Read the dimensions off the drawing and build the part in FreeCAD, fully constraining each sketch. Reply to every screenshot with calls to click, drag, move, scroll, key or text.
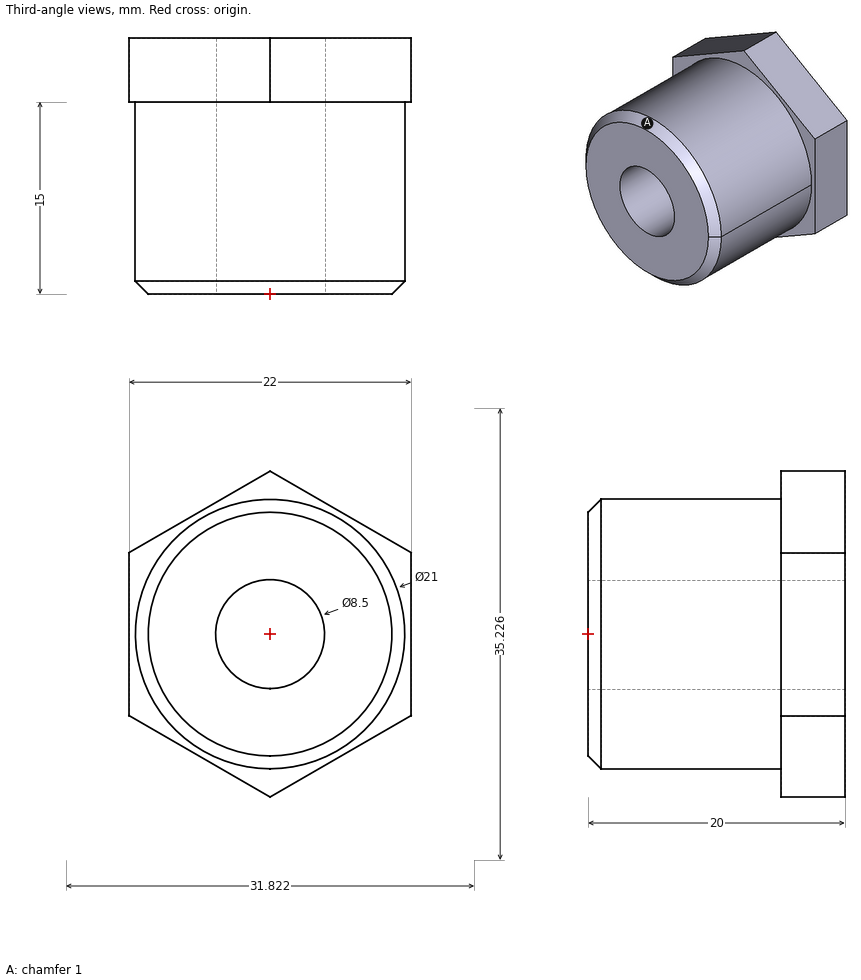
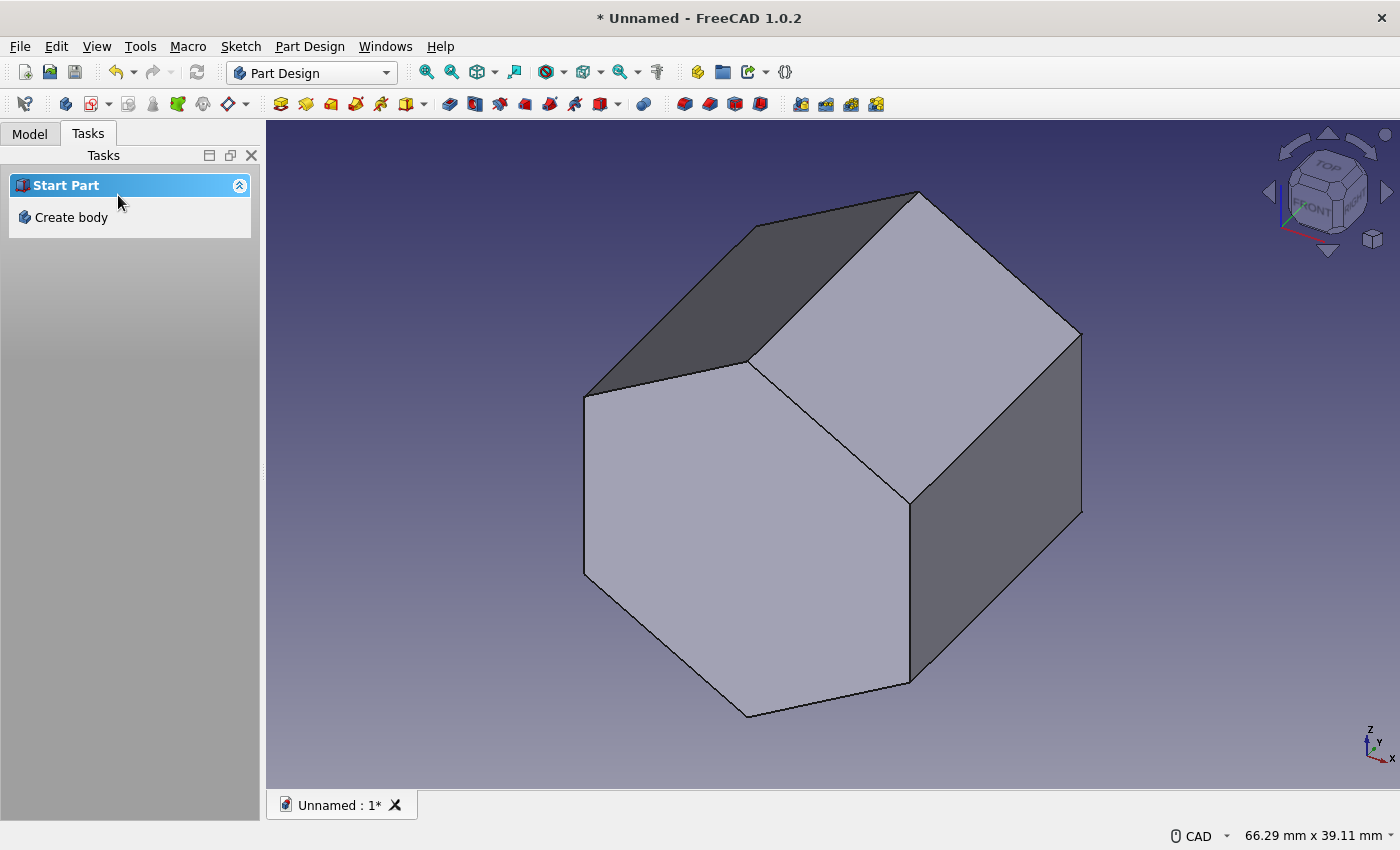
click(747, 538)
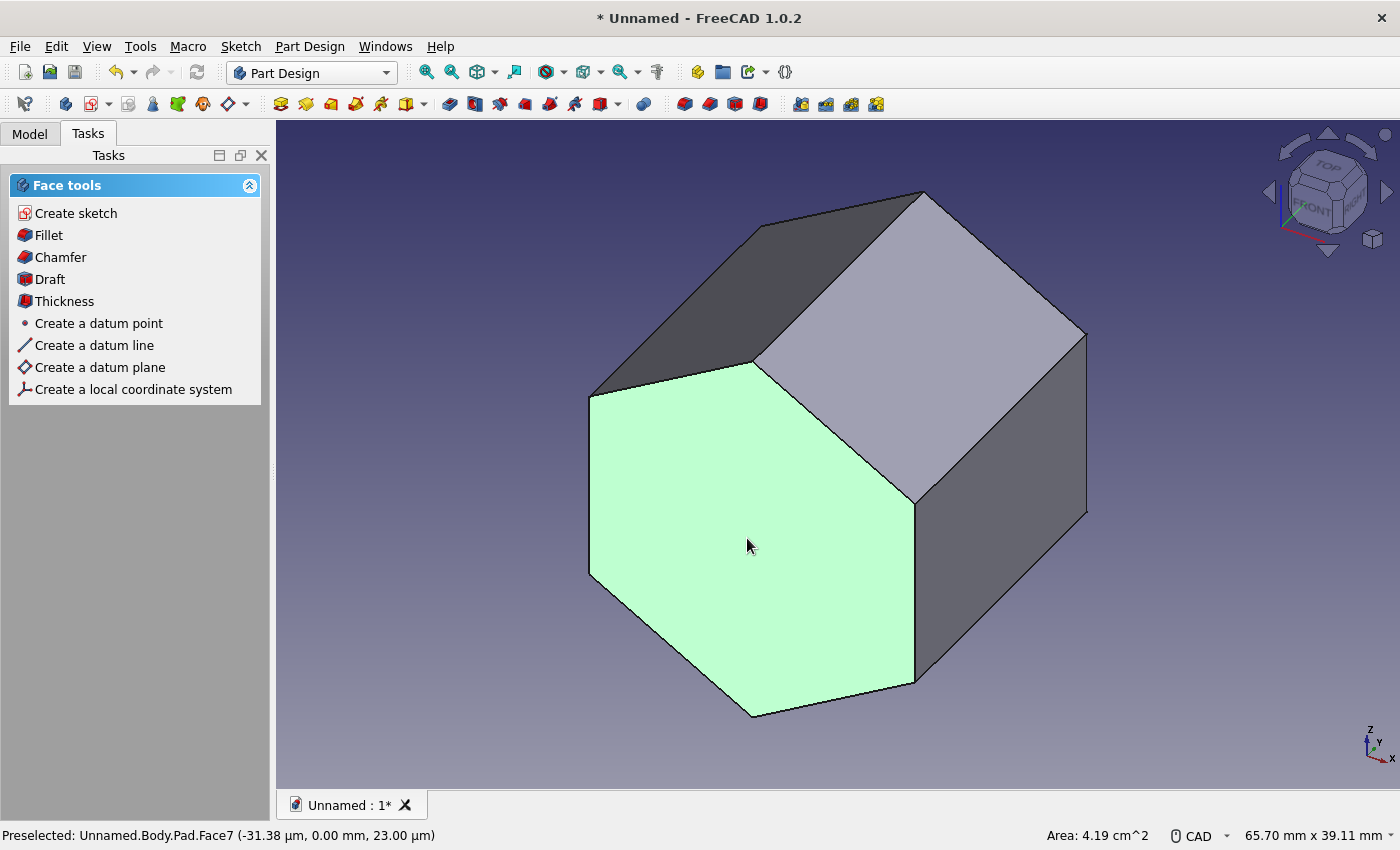
click(90, 104)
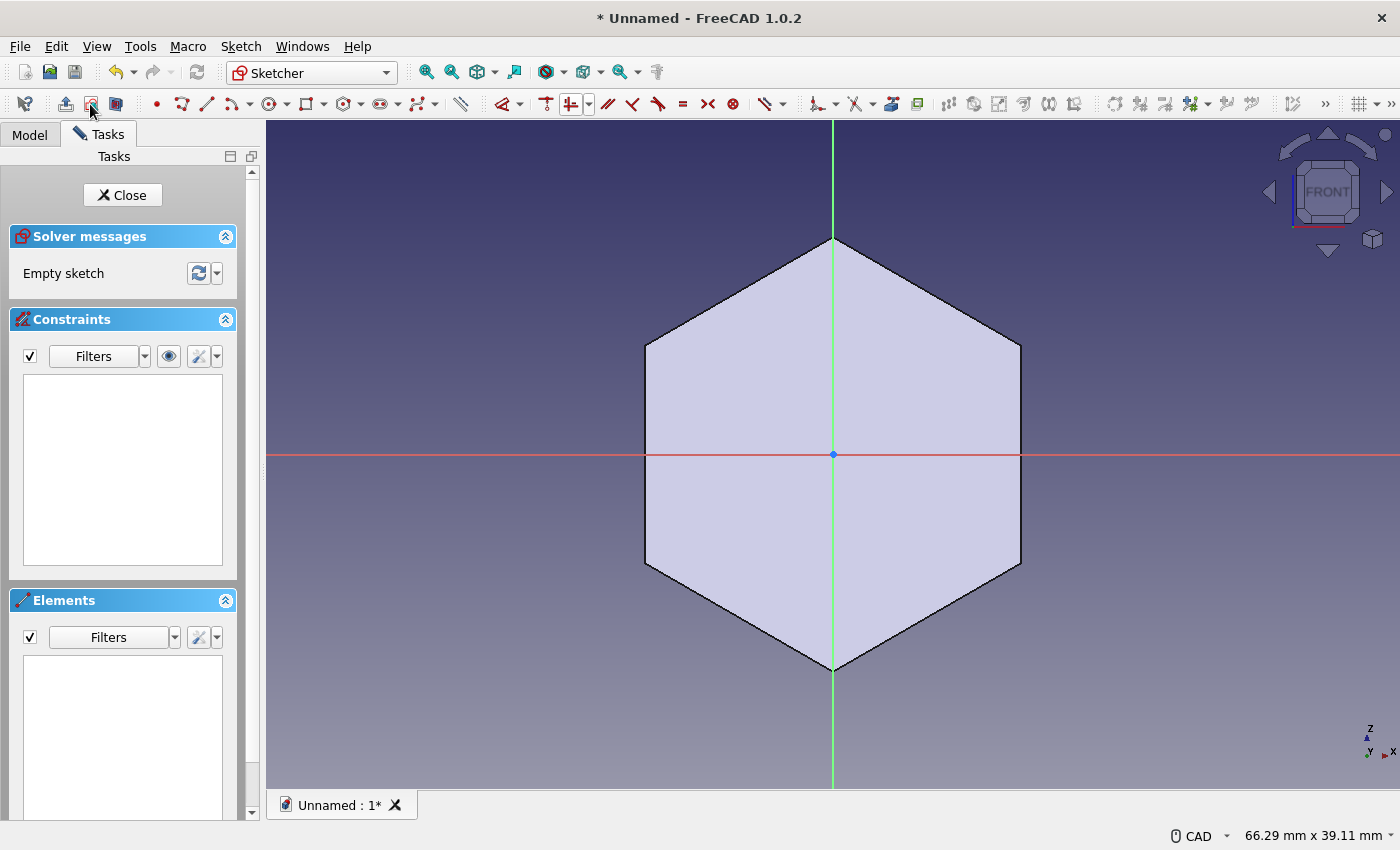
scroll(625, 454, down, 2)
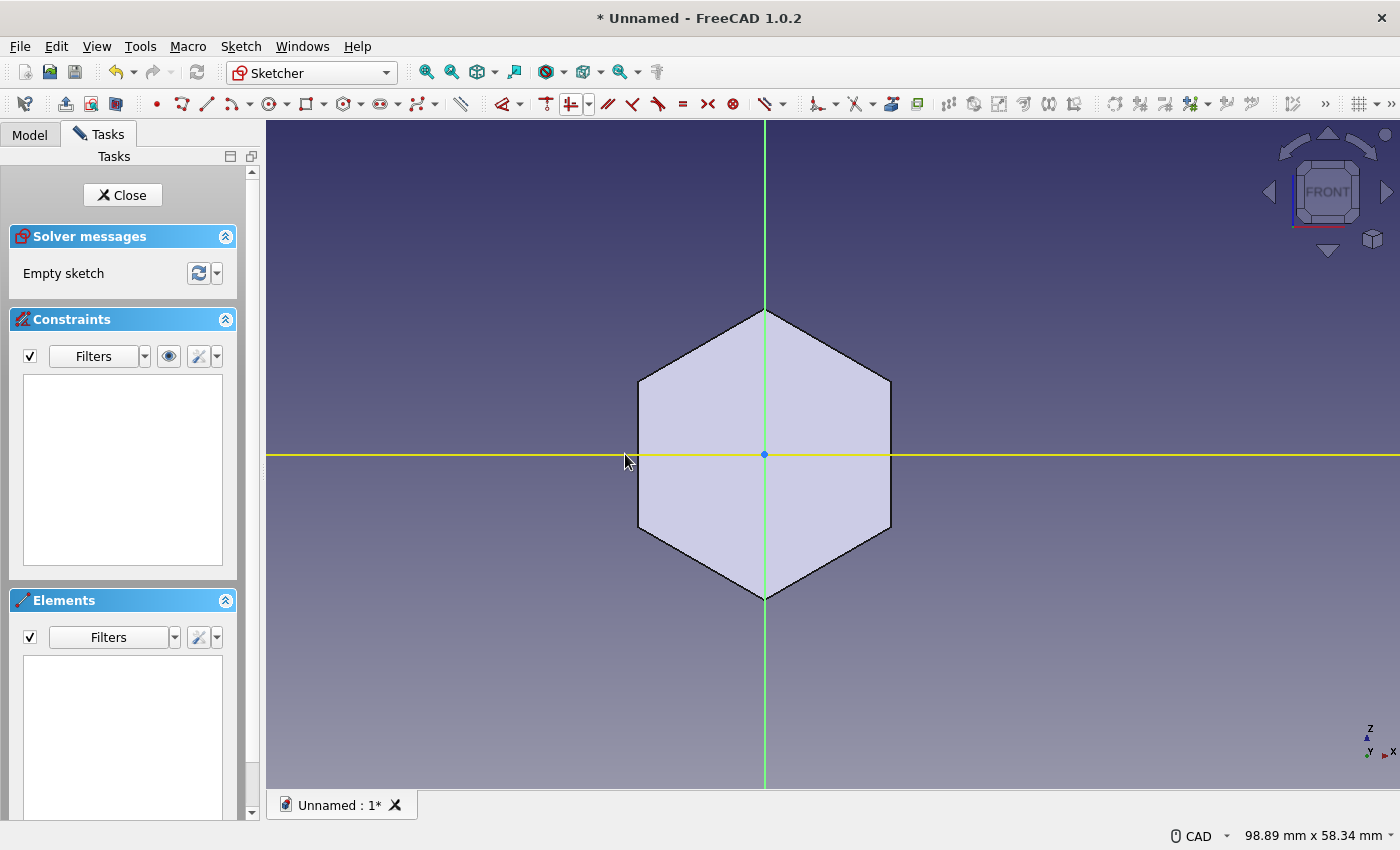
key(g)
key(v)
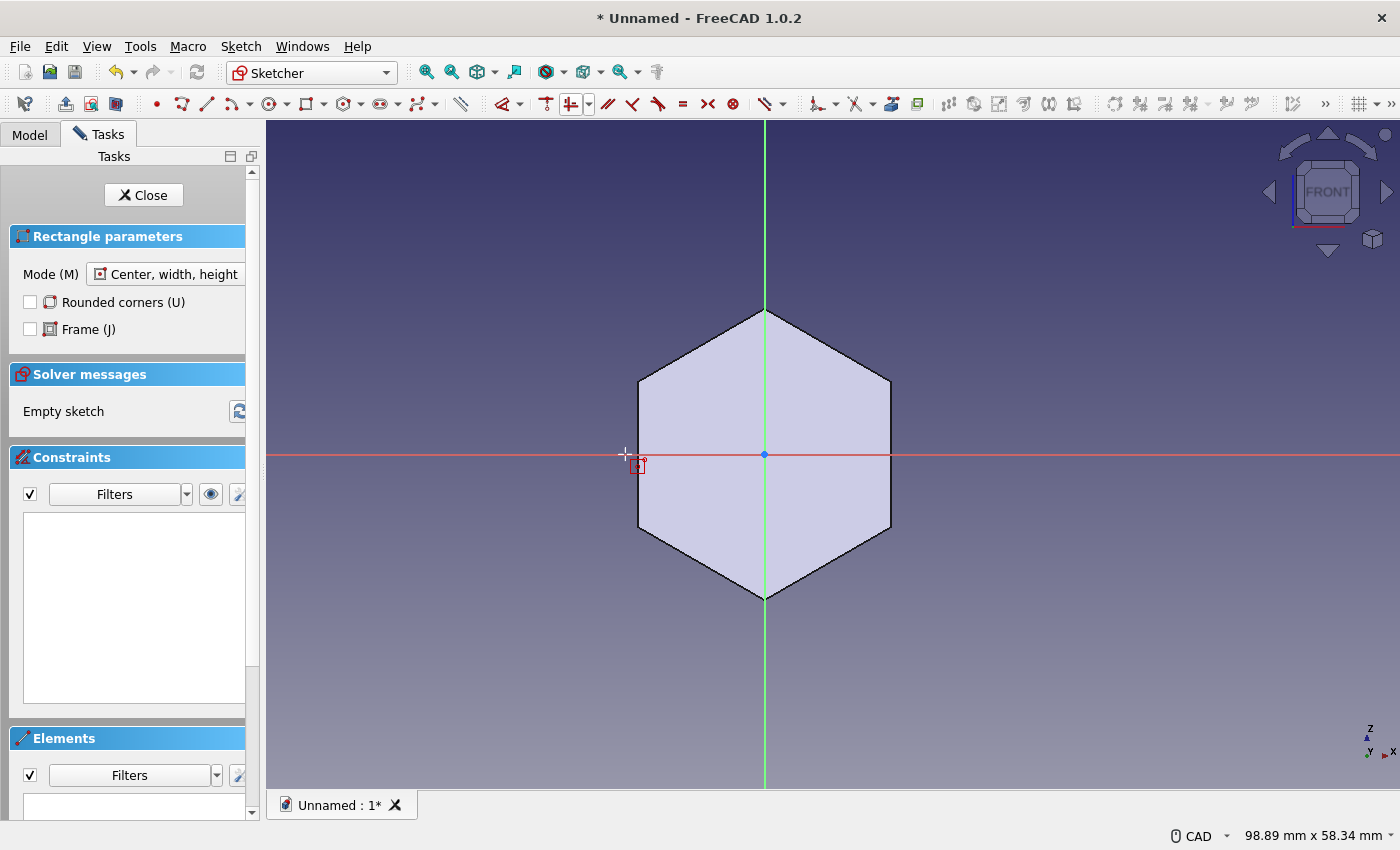
click(765, 455)
move(947, 253)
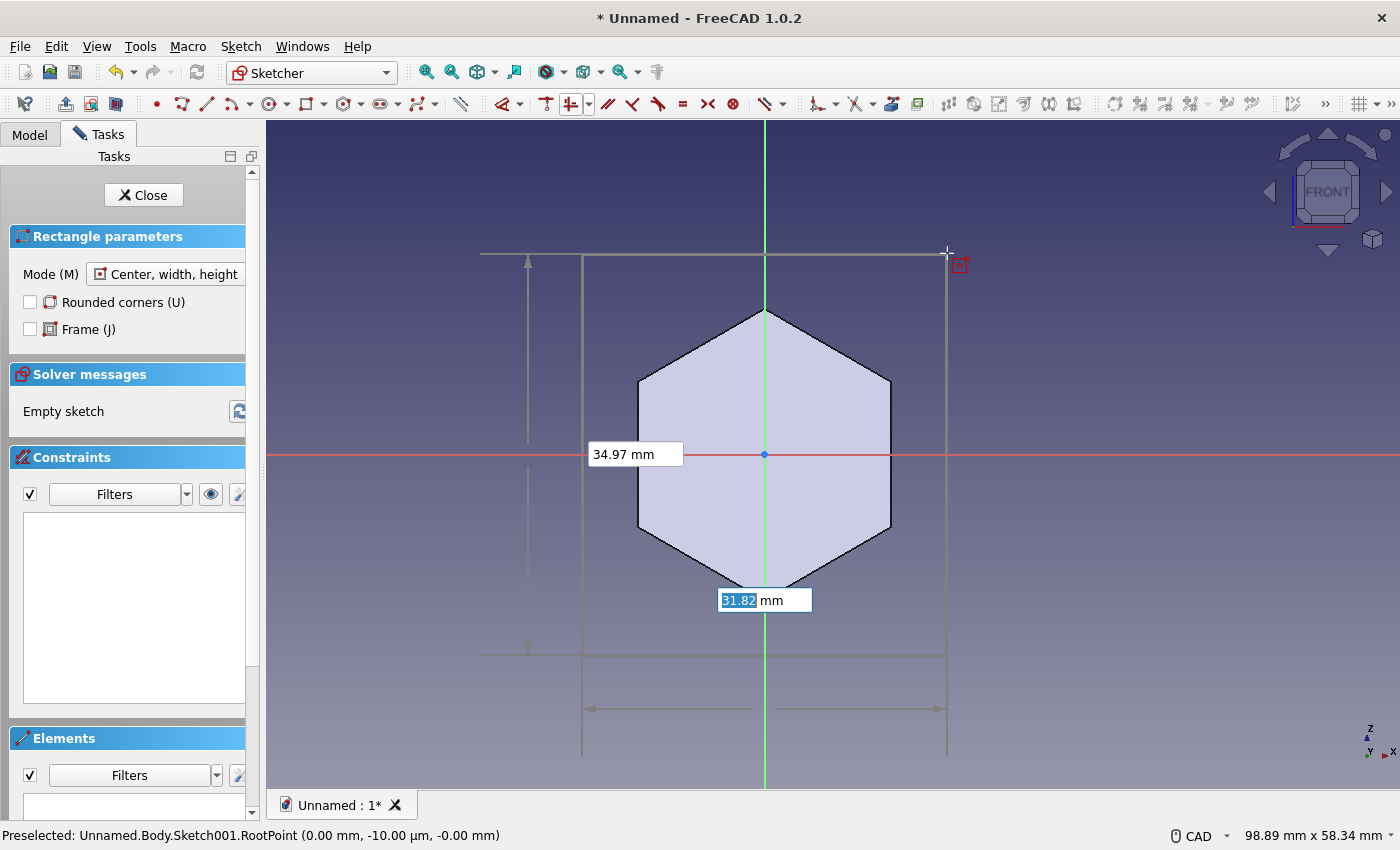
text(31.822)
key(Tab)
text(35.226)
key(Return)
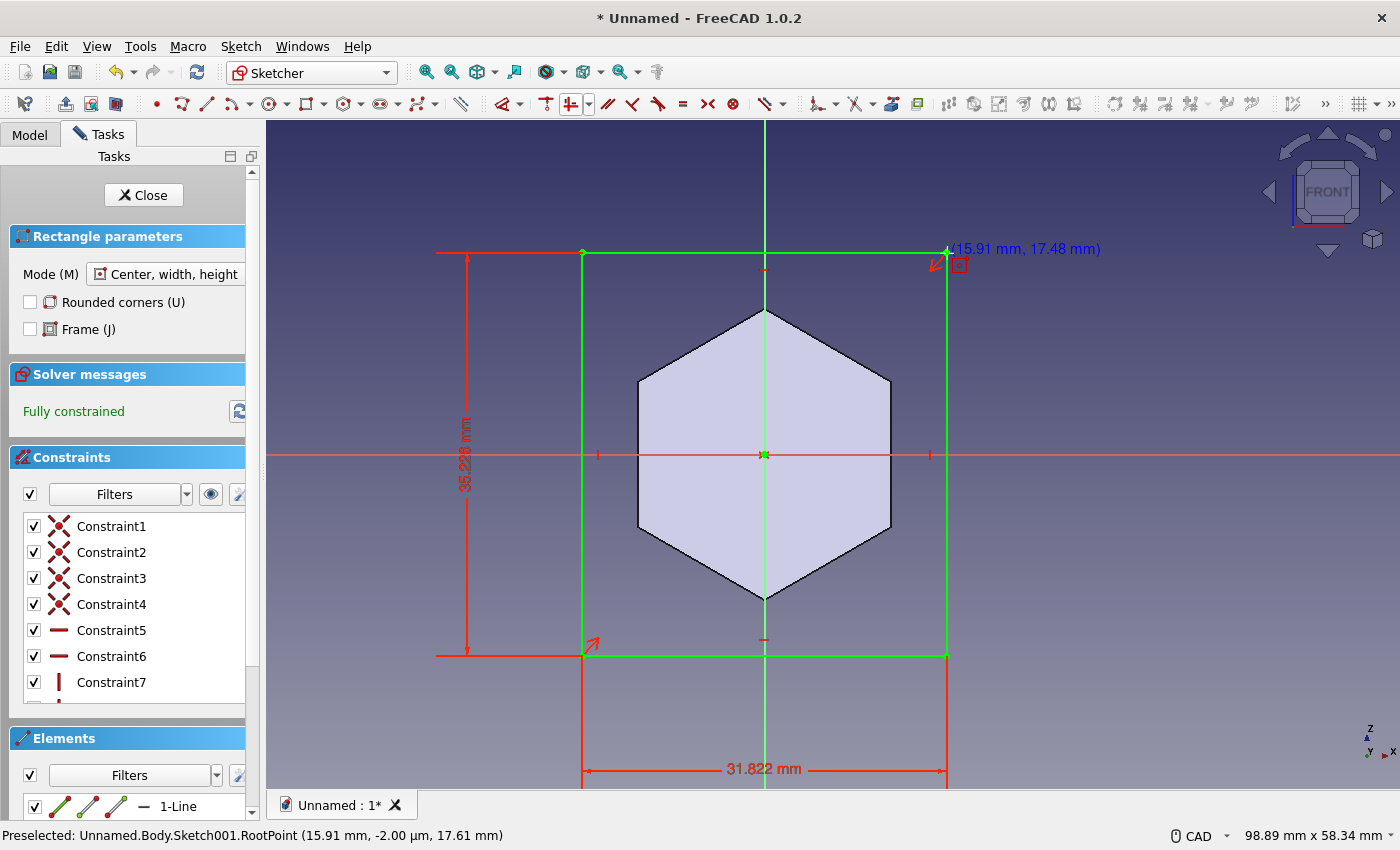
key(g)
key(c)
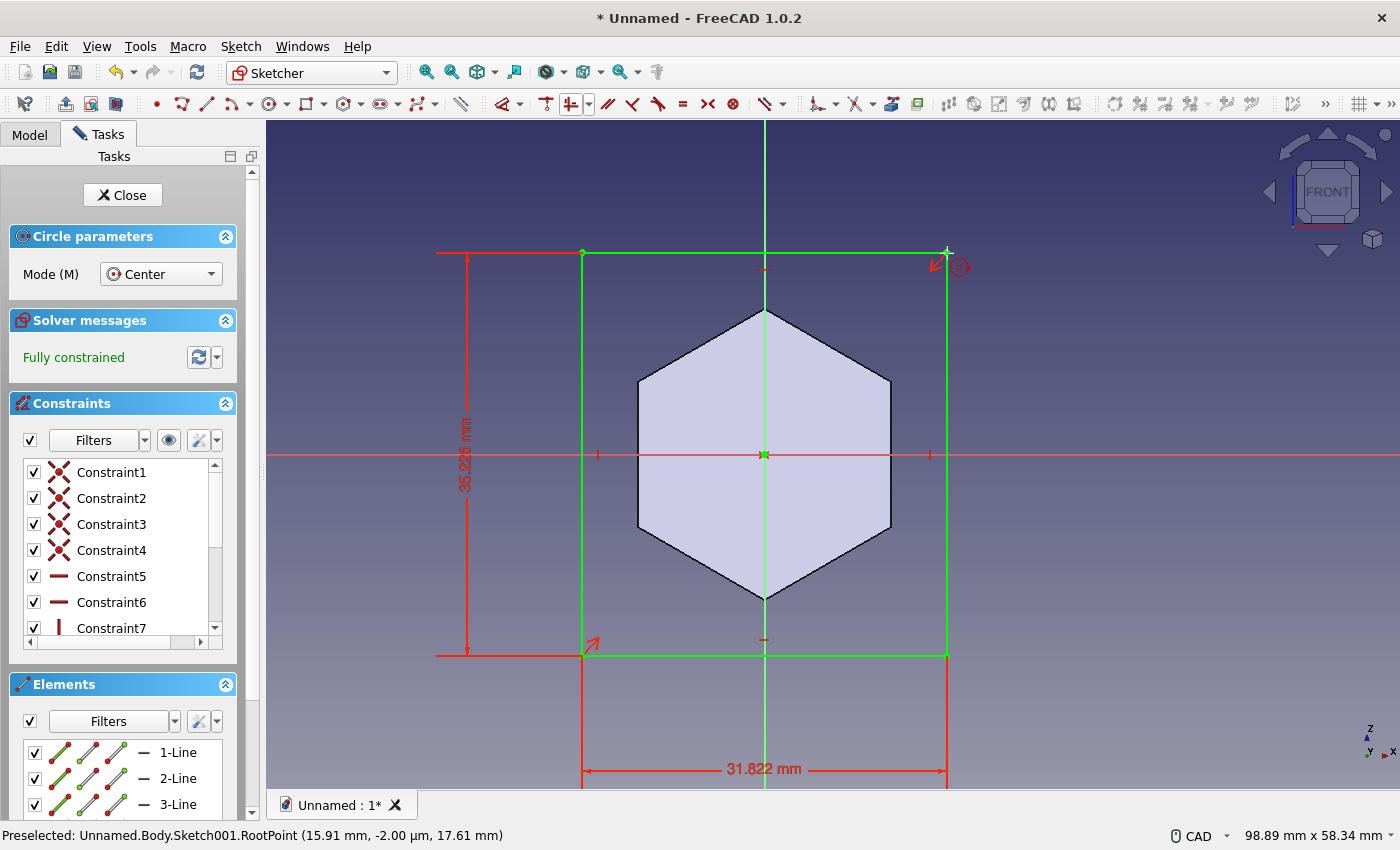
click(765, 455)
move(850, 369)